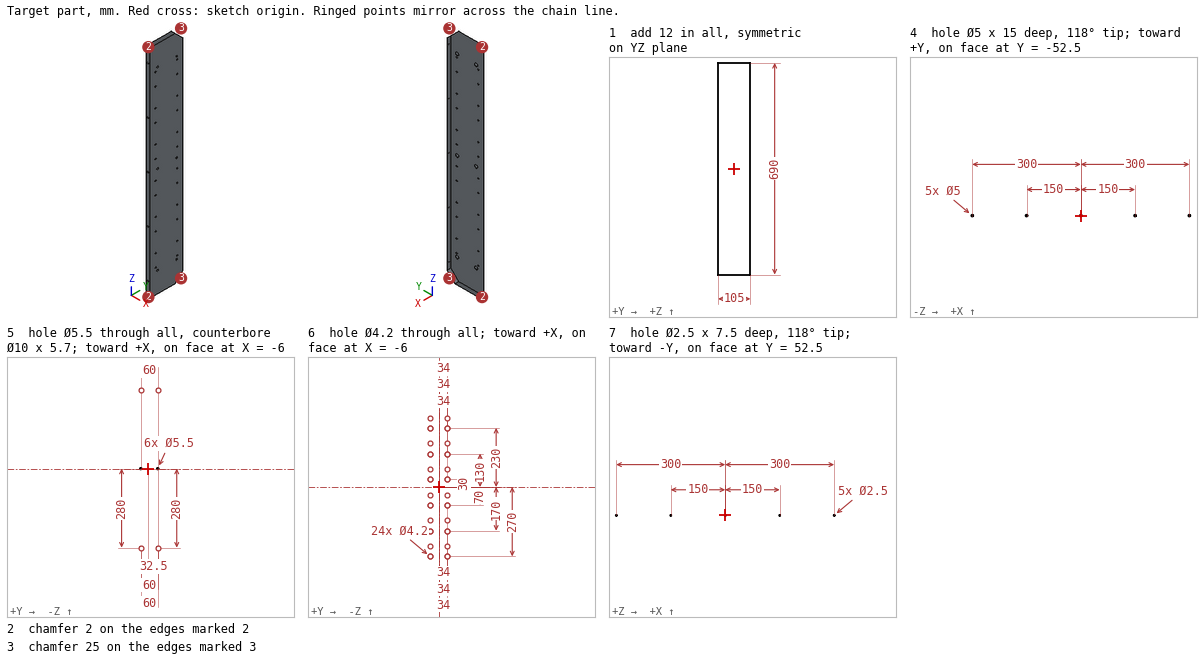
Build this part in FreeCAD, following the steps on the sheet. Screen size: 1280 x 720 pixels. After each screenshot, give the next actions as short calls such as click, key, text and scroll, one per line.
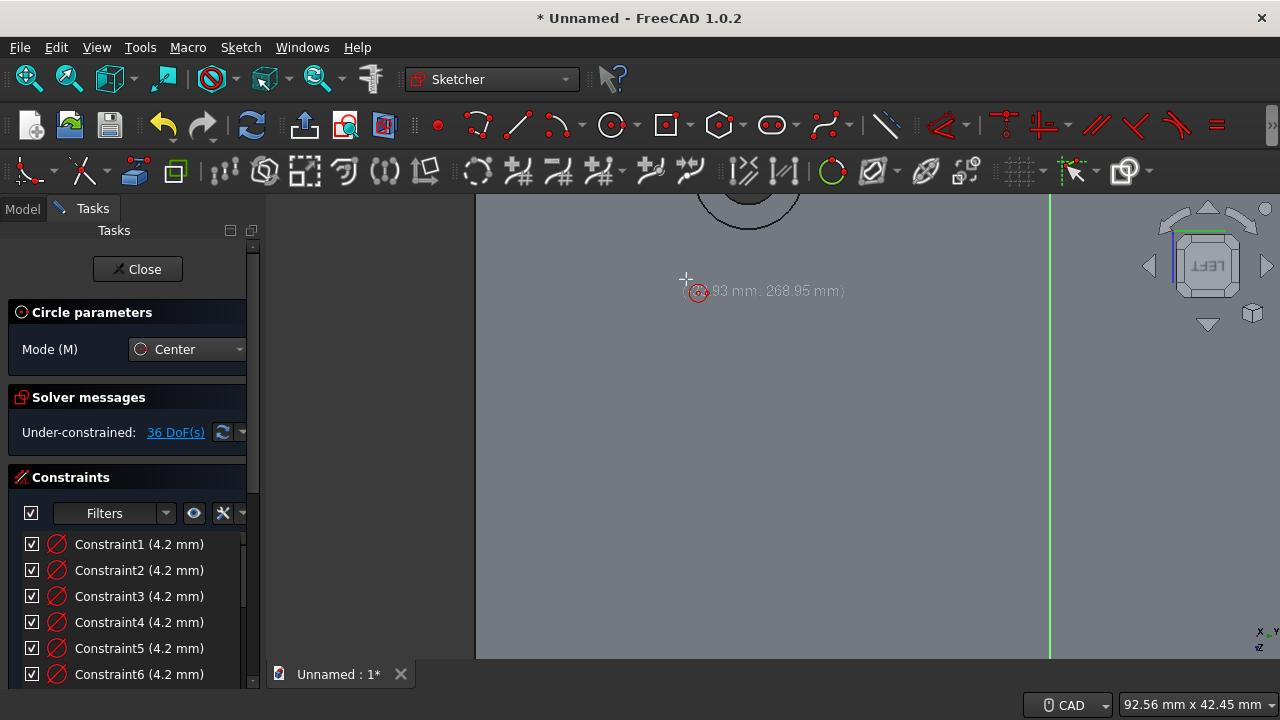
scroll(686, 279, down, 15)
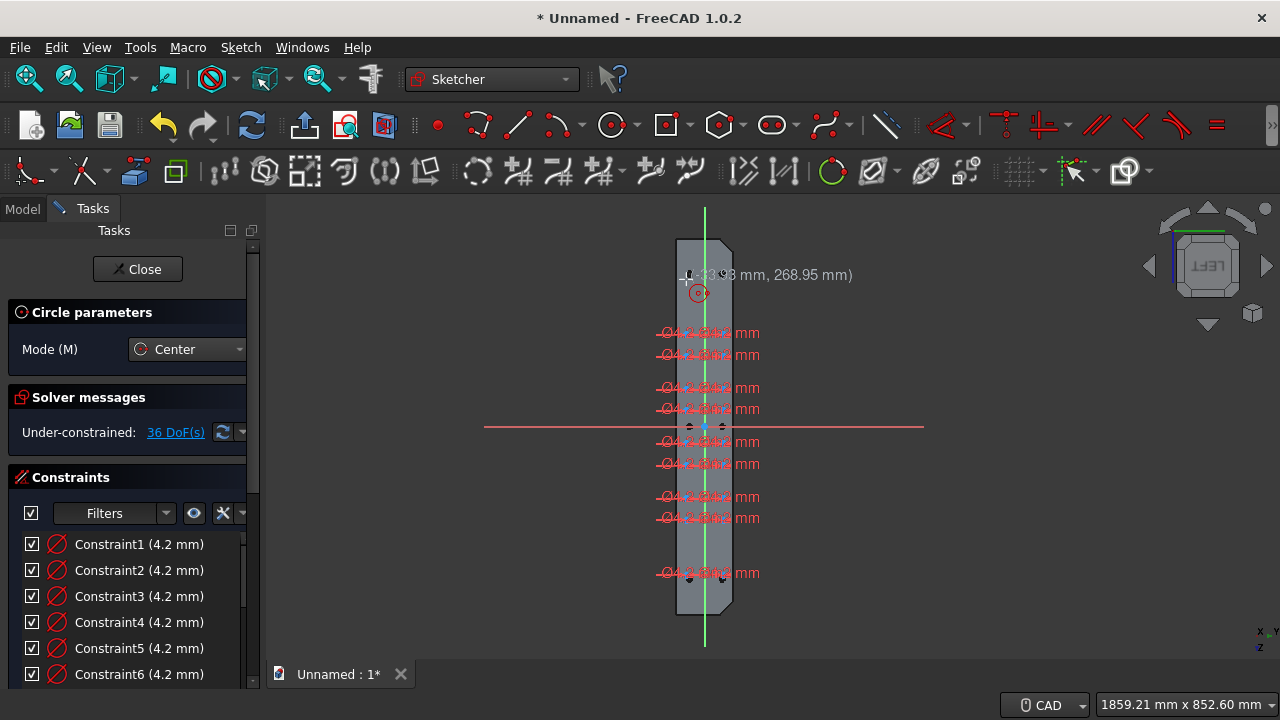
click(686, 279)
move(687, 279)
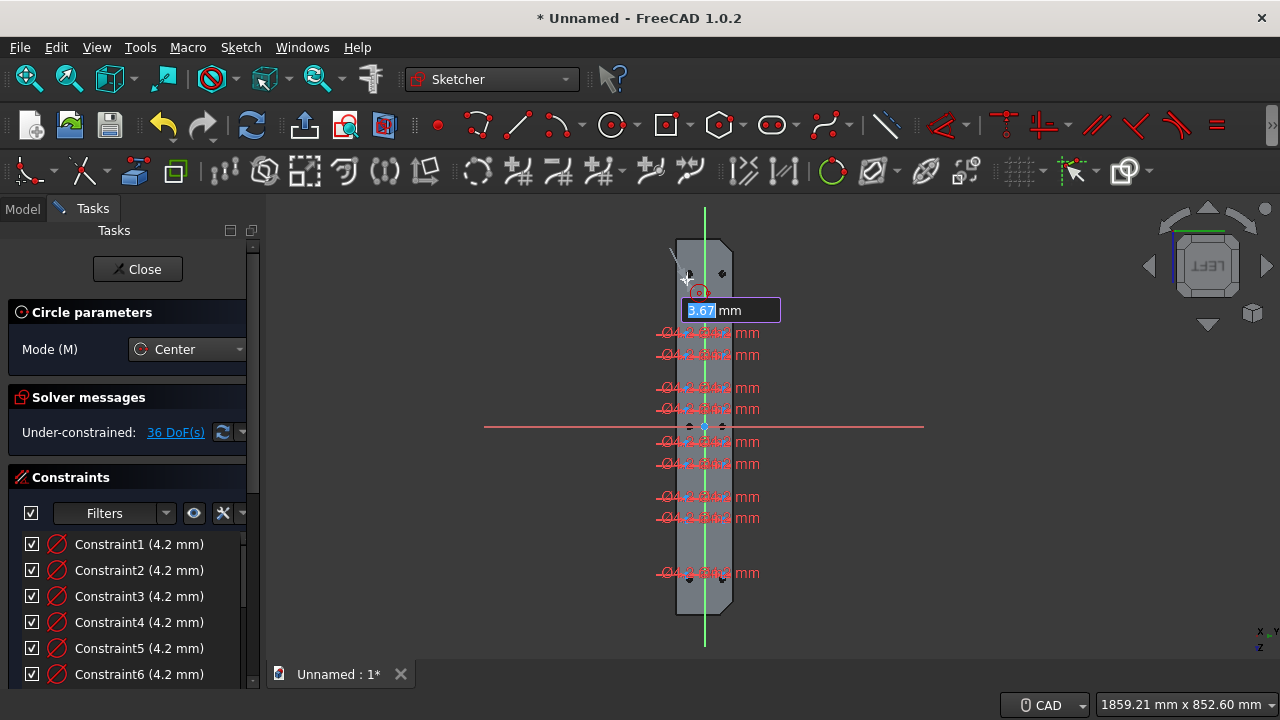
text(4.2)
key(Return)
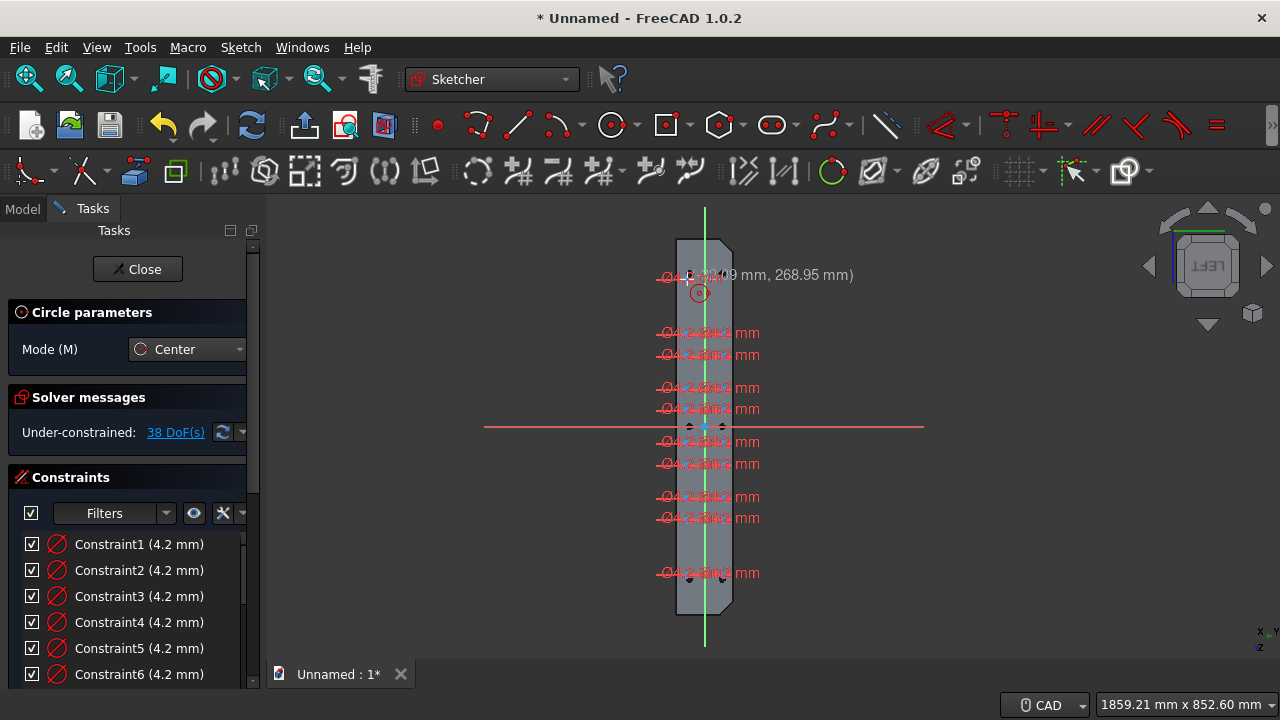
scroll(723, 279, up, 15)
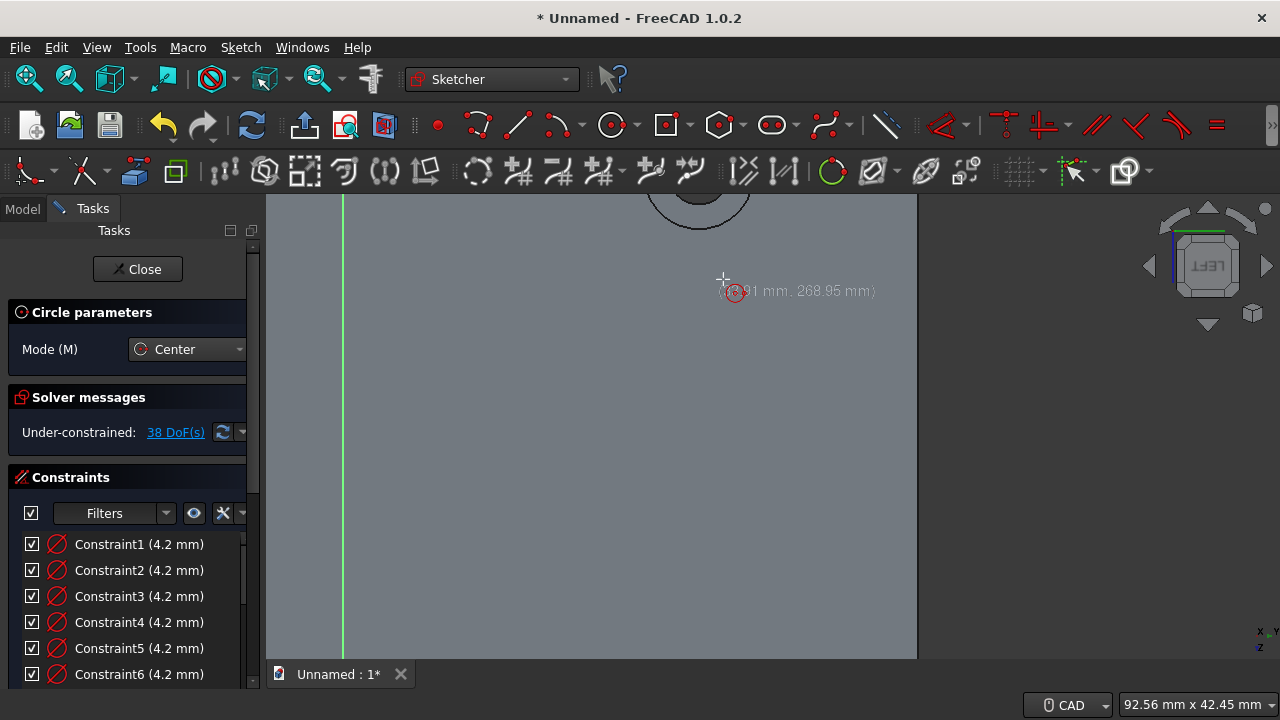
scroll(723, 279, down, 15)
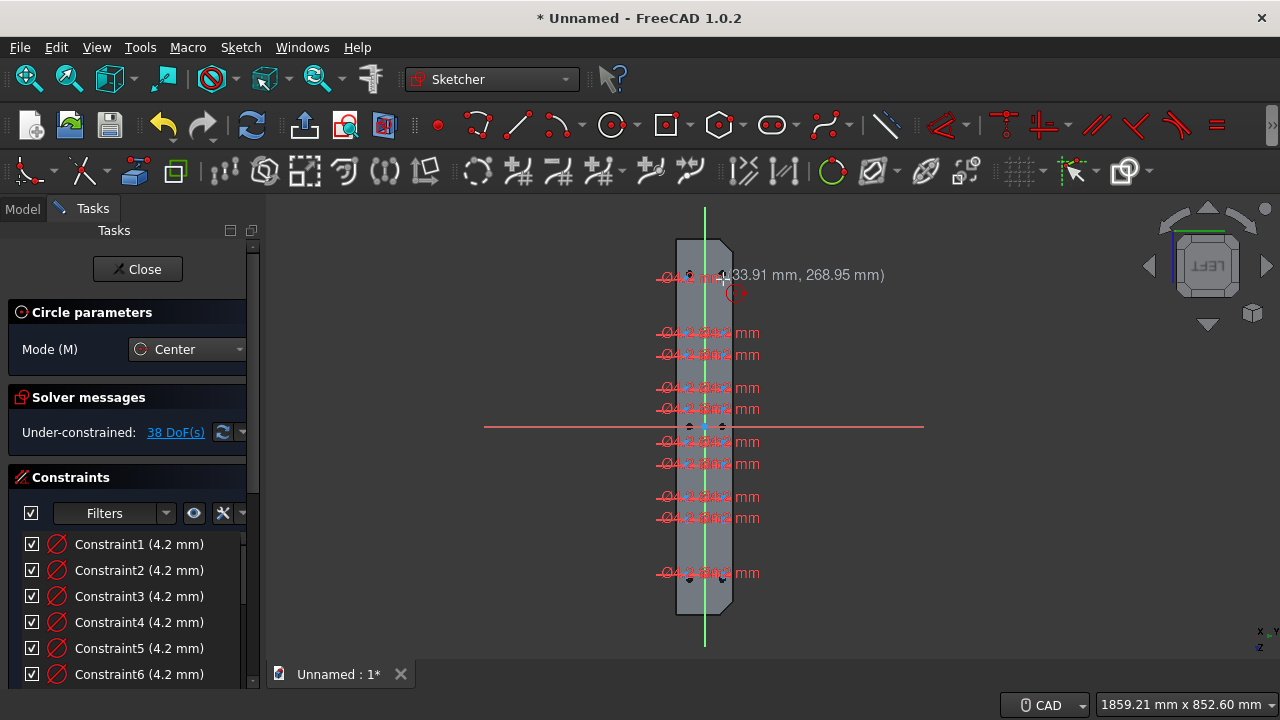
click(723, 279)
move(724, 279)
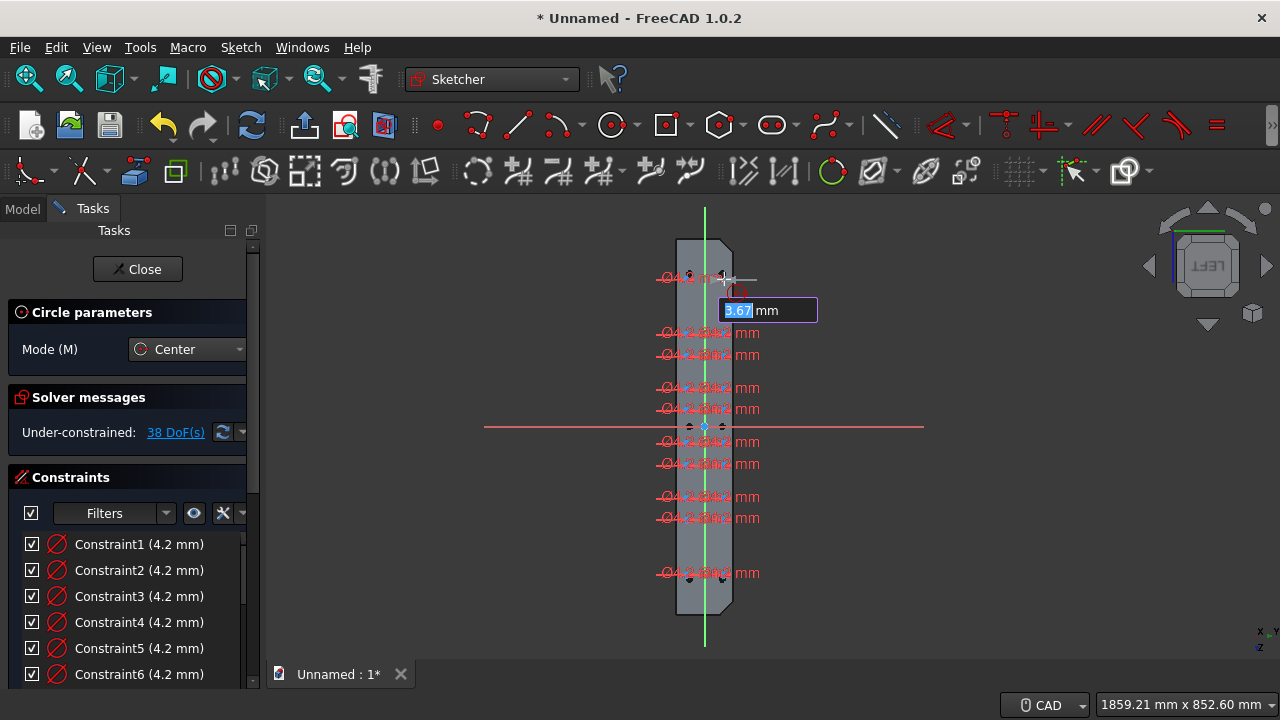
text(4.2)
key(Return)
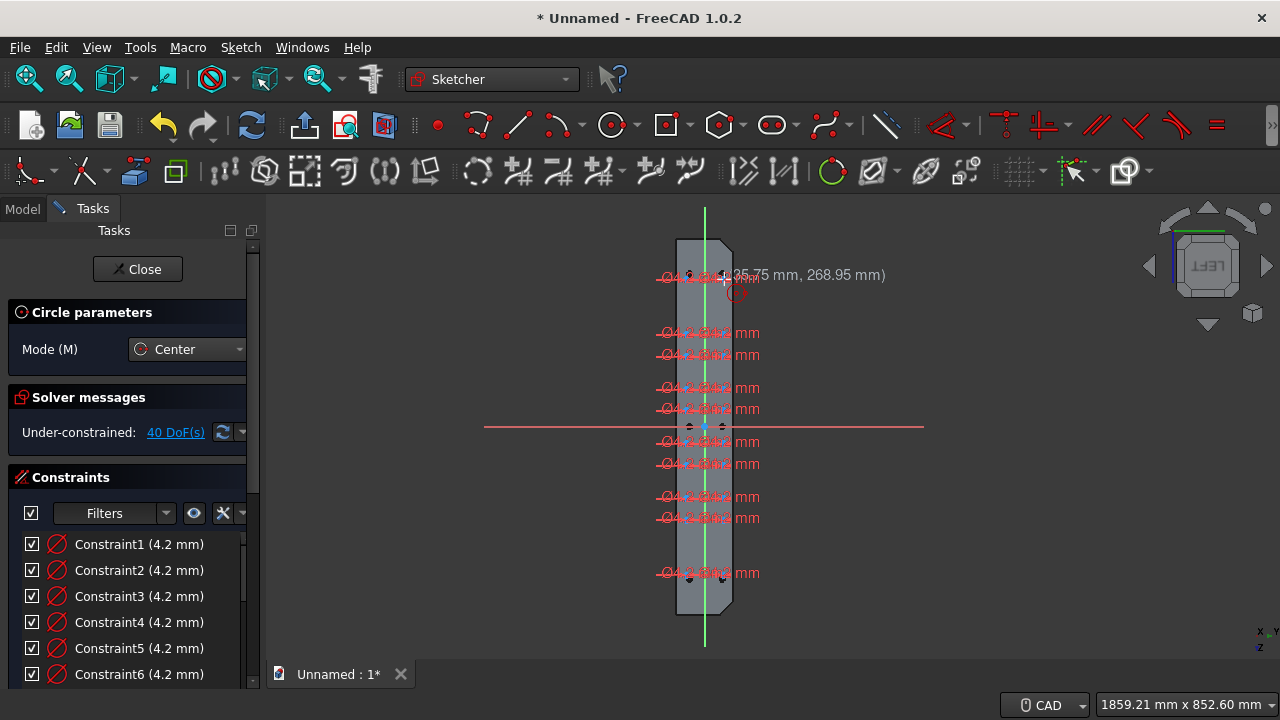
scroll(723, 301, up, 15)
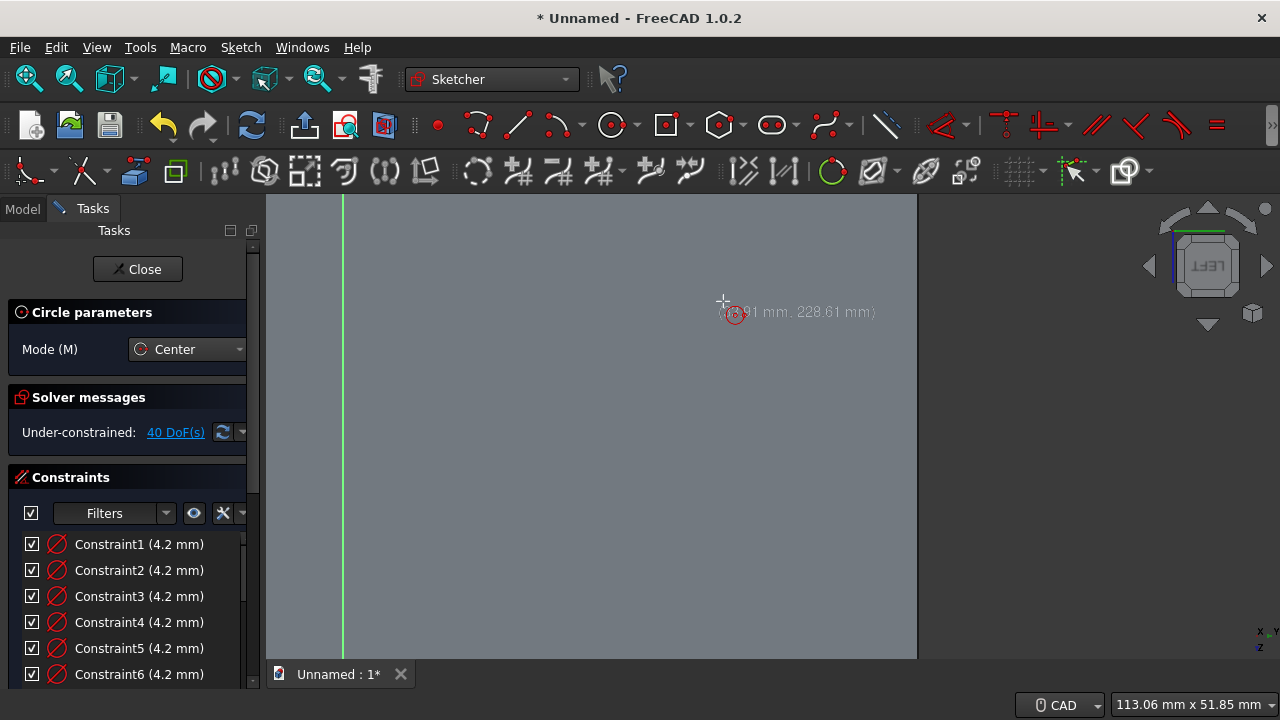
scroll(723, 301, down, 15)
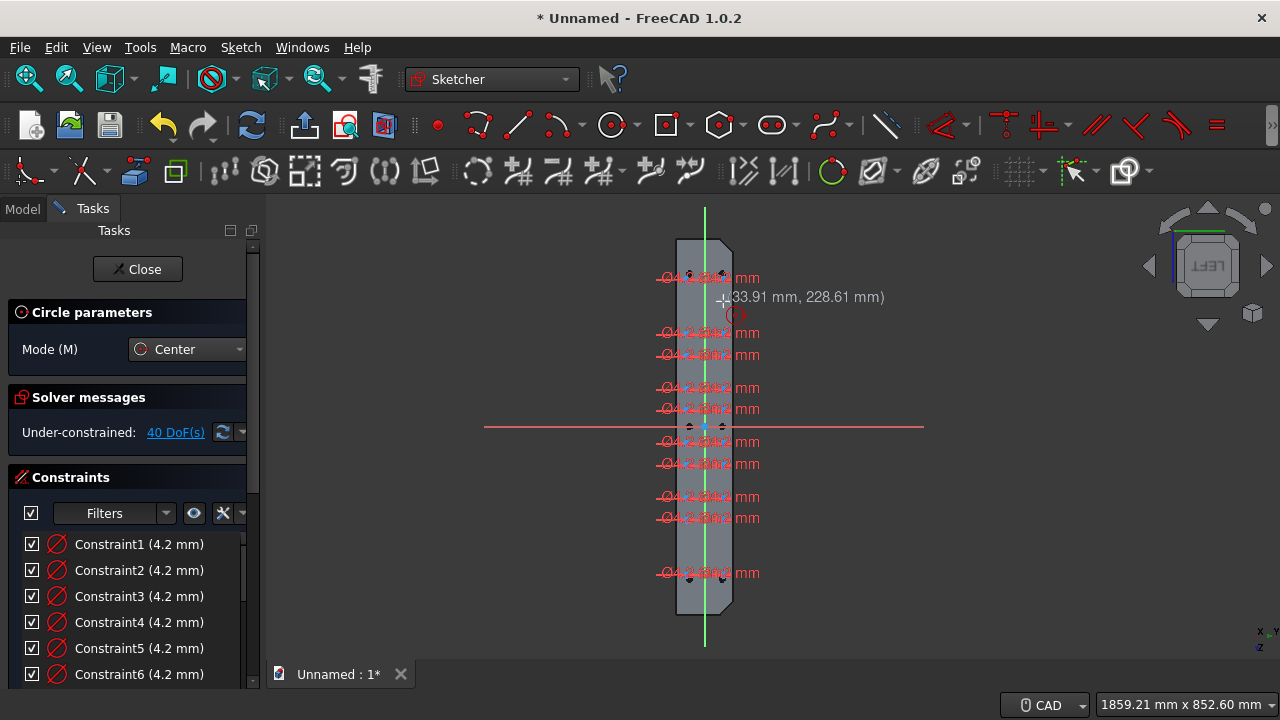
click(723, 301)
move(724, 300)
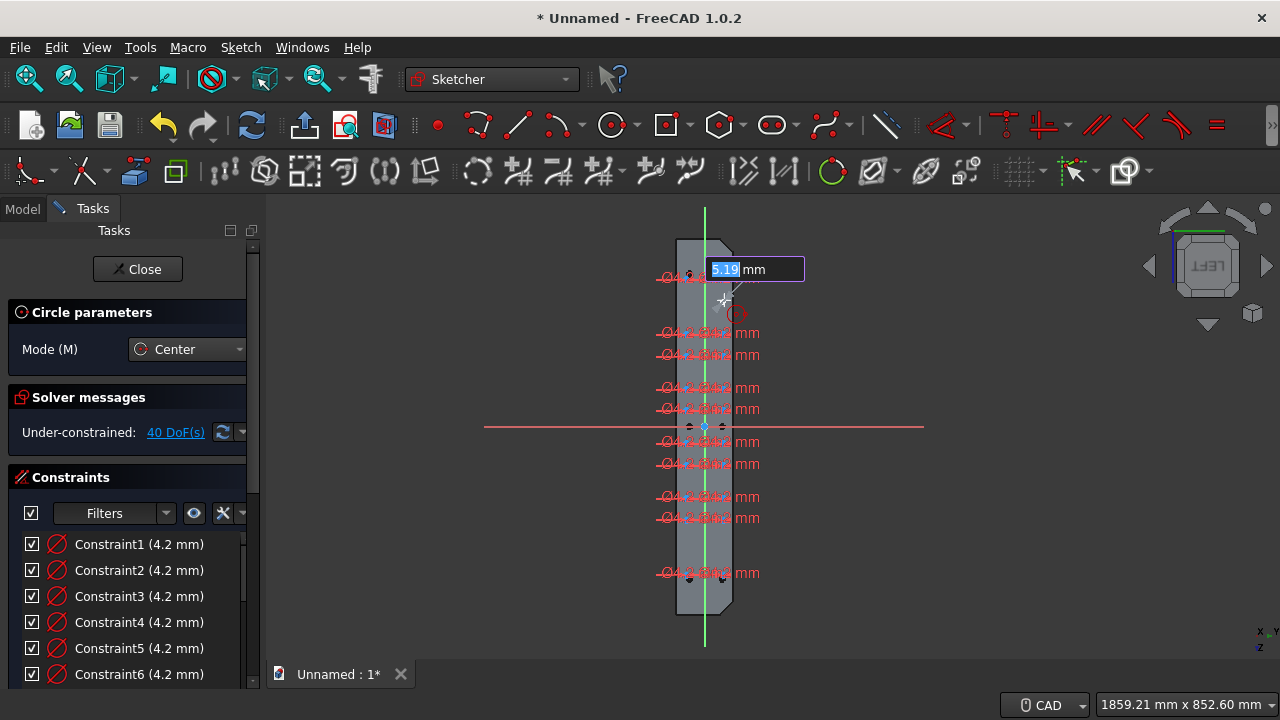
text(4.2)
key(Return)